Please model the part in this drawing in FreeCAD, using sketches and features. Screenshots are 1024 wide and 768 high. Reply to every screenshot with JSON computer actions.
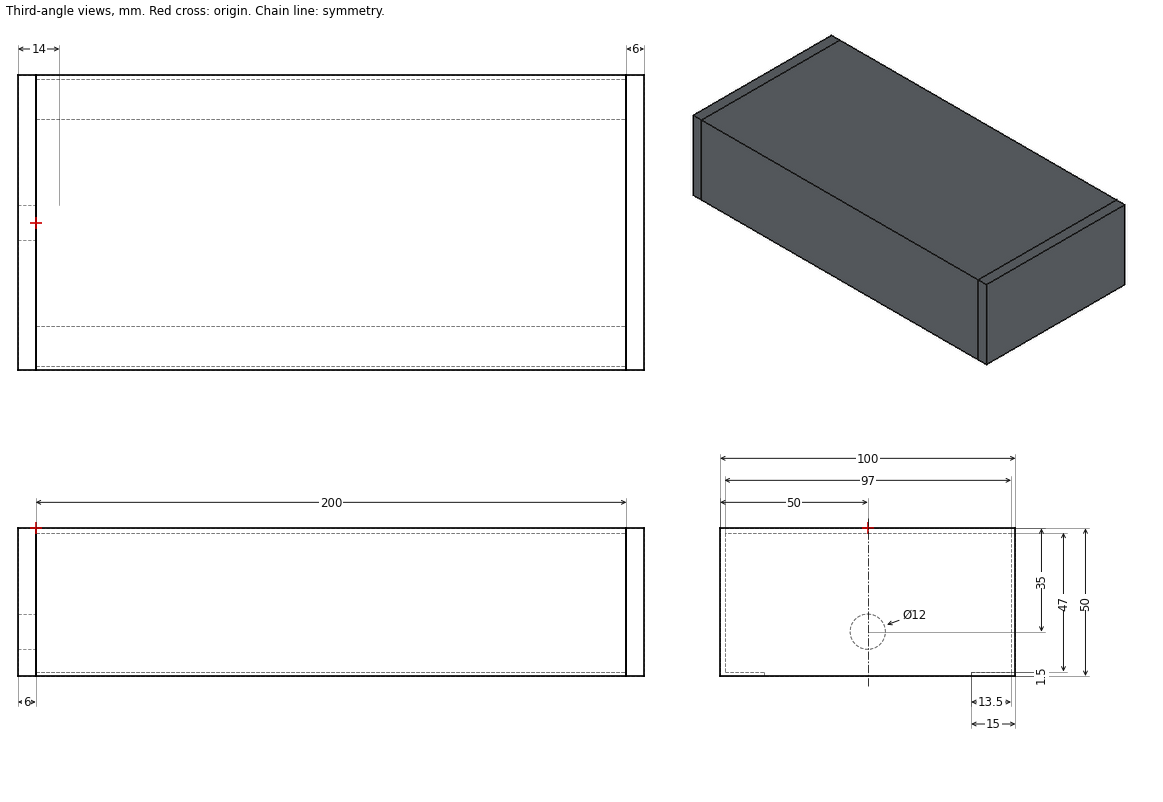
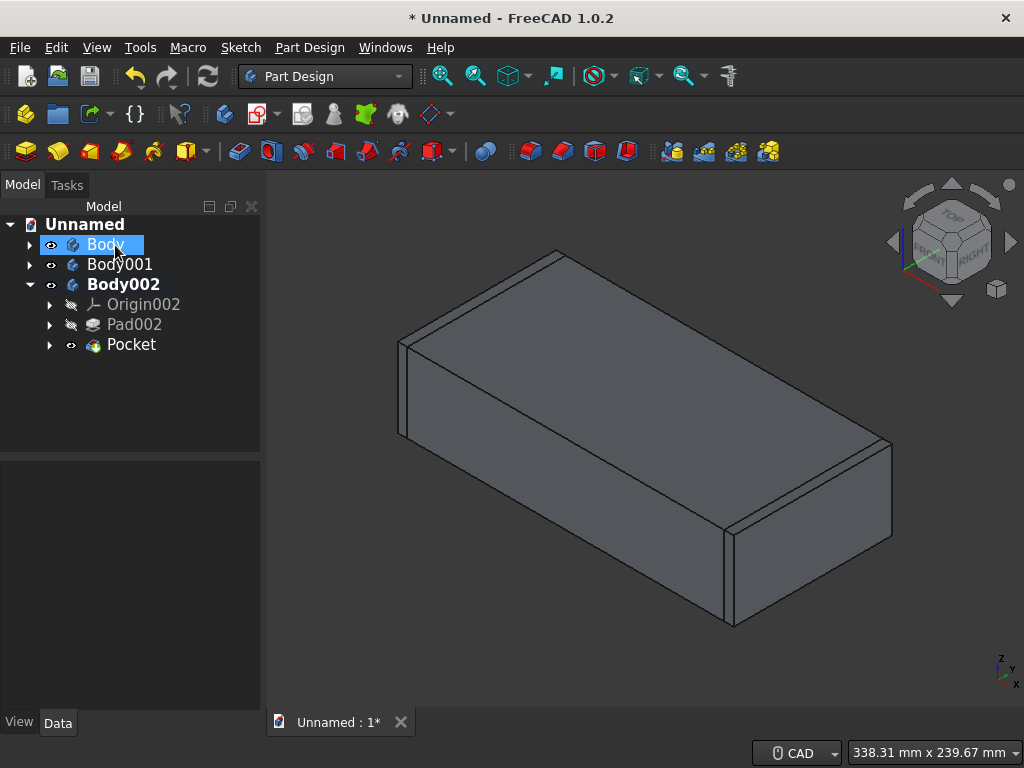
{"action": "left_click", "coordinate": [444, 76]}